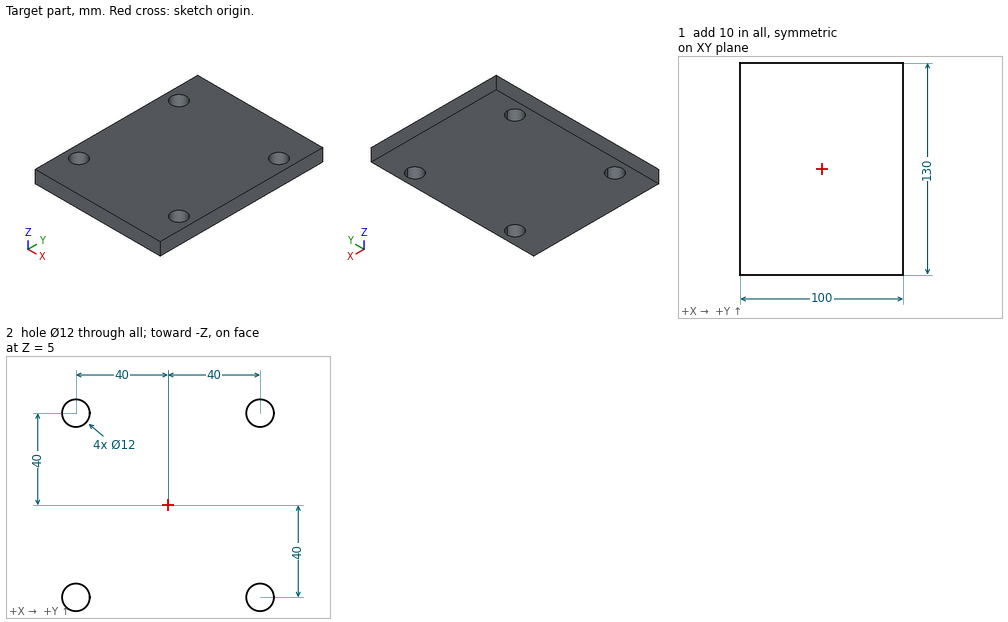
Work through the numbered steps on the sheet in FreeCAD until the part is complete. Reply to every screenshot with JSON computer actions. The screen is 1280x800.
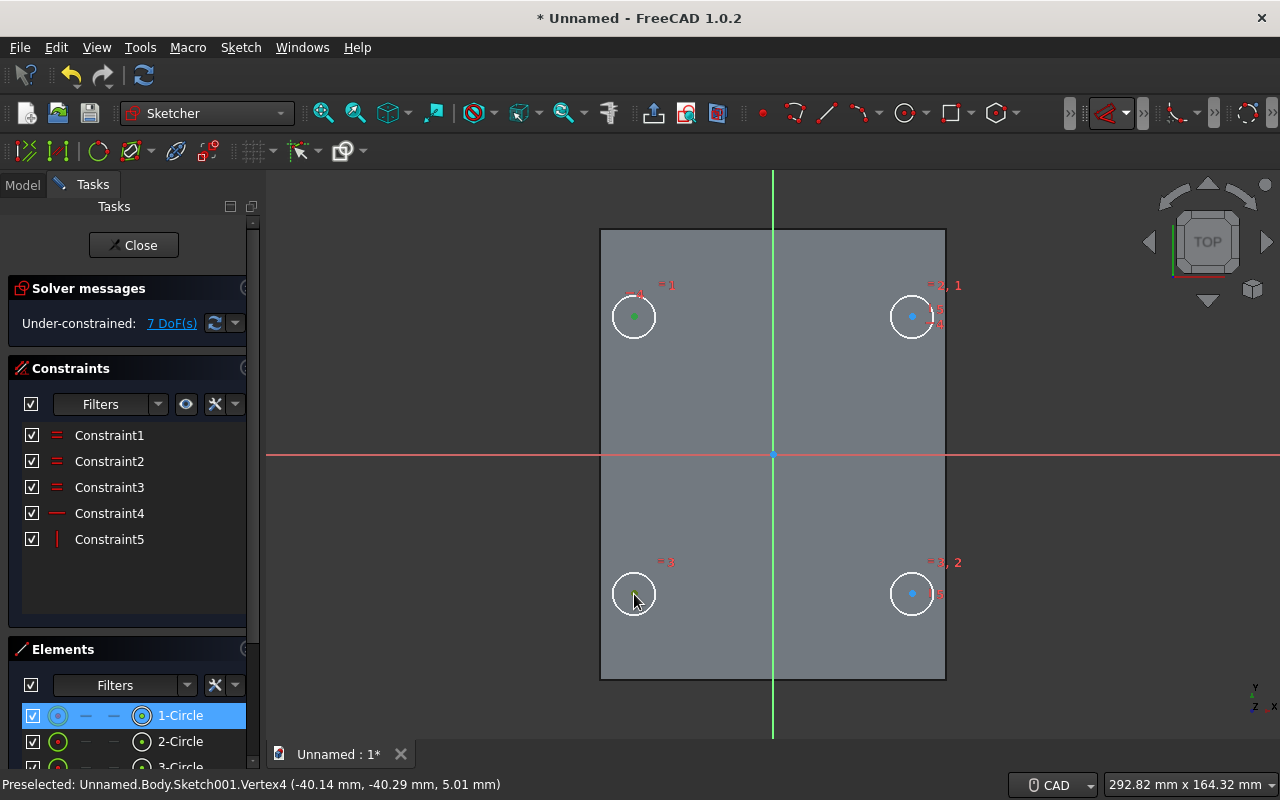
{"action": "key", "text": "v"}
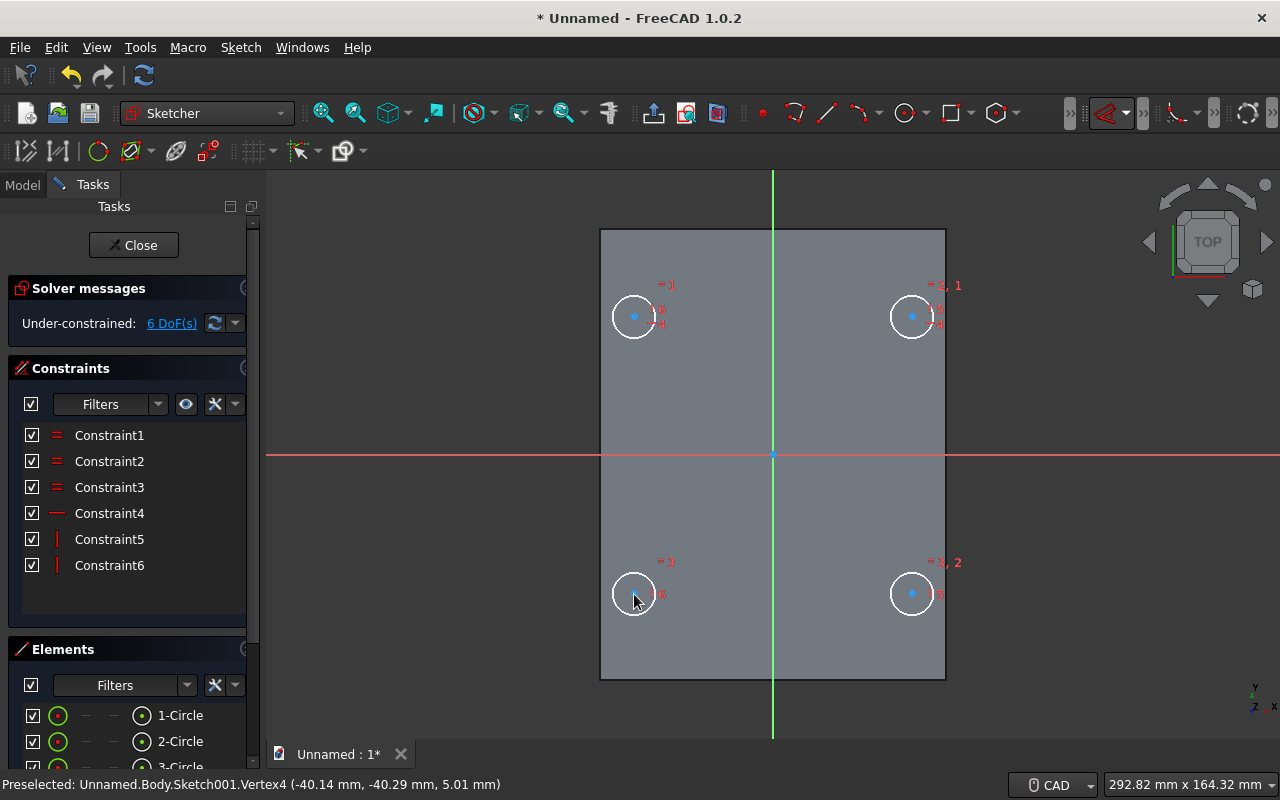
{"action": "left_click", "coordinate": [912, 594]}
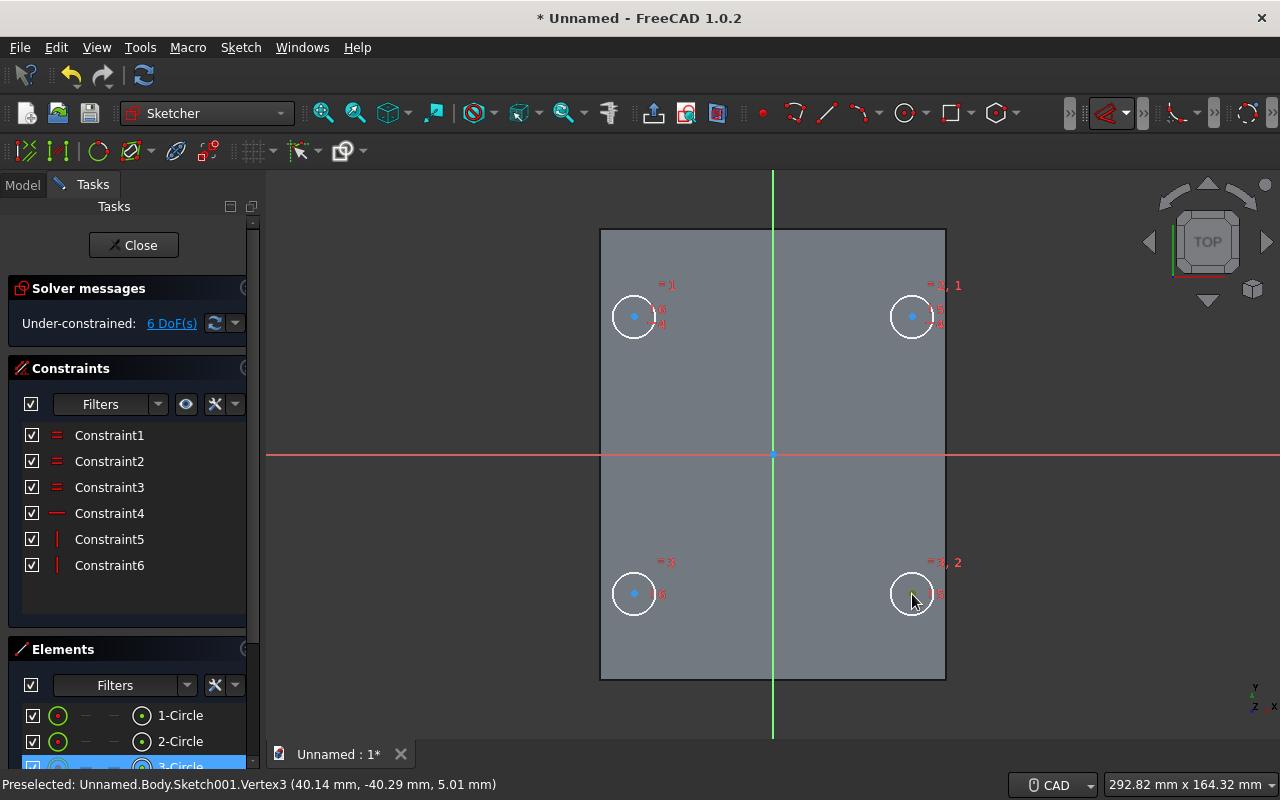
{"action": "left_click", "coordinate": [634, 594]}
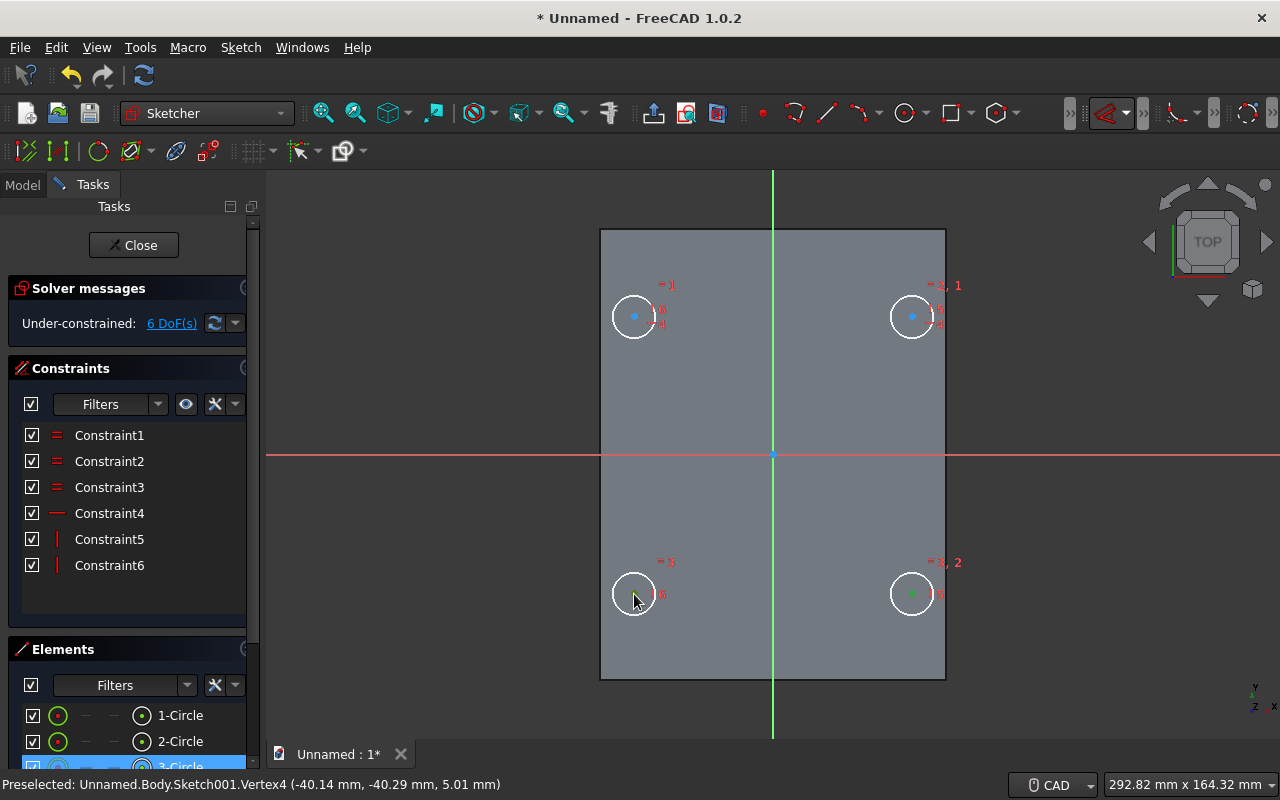
{"action": "key", "text": "h"}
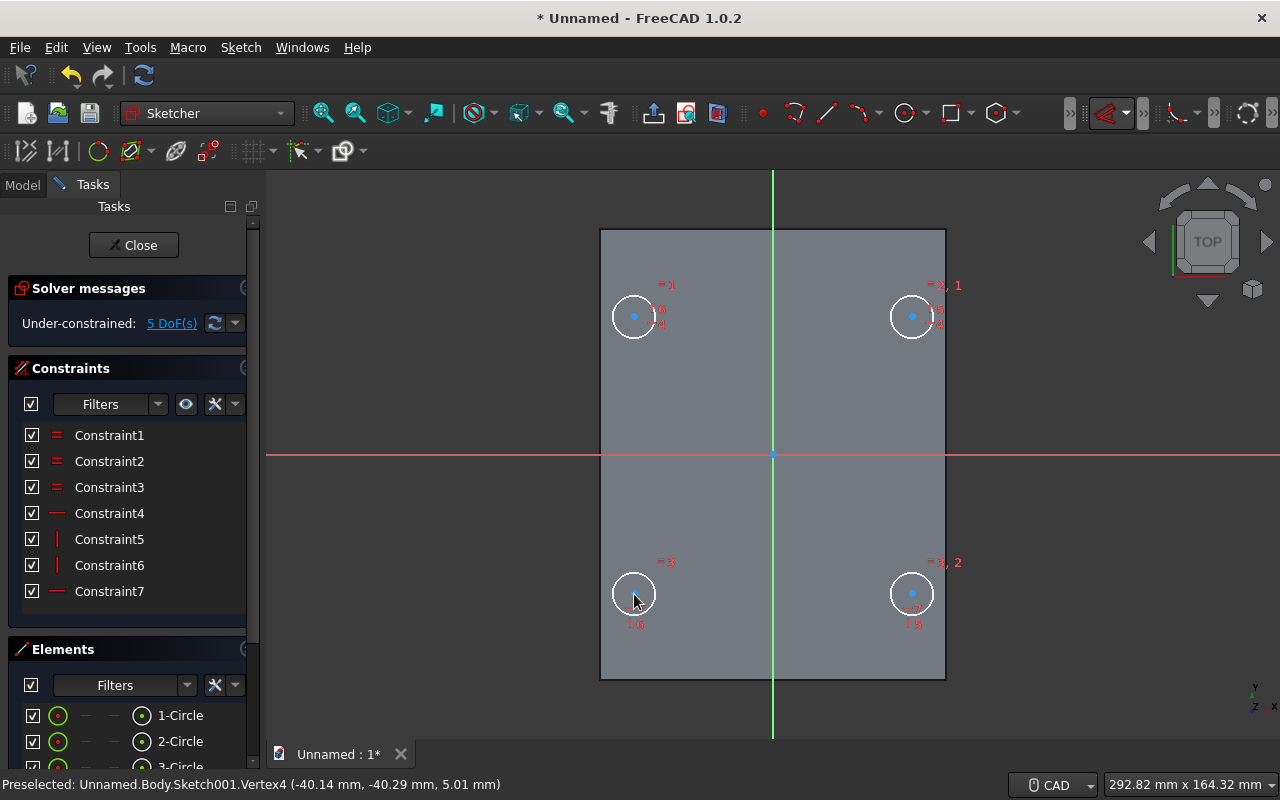
{"action": "left_click", "coordinate": [619, 302]}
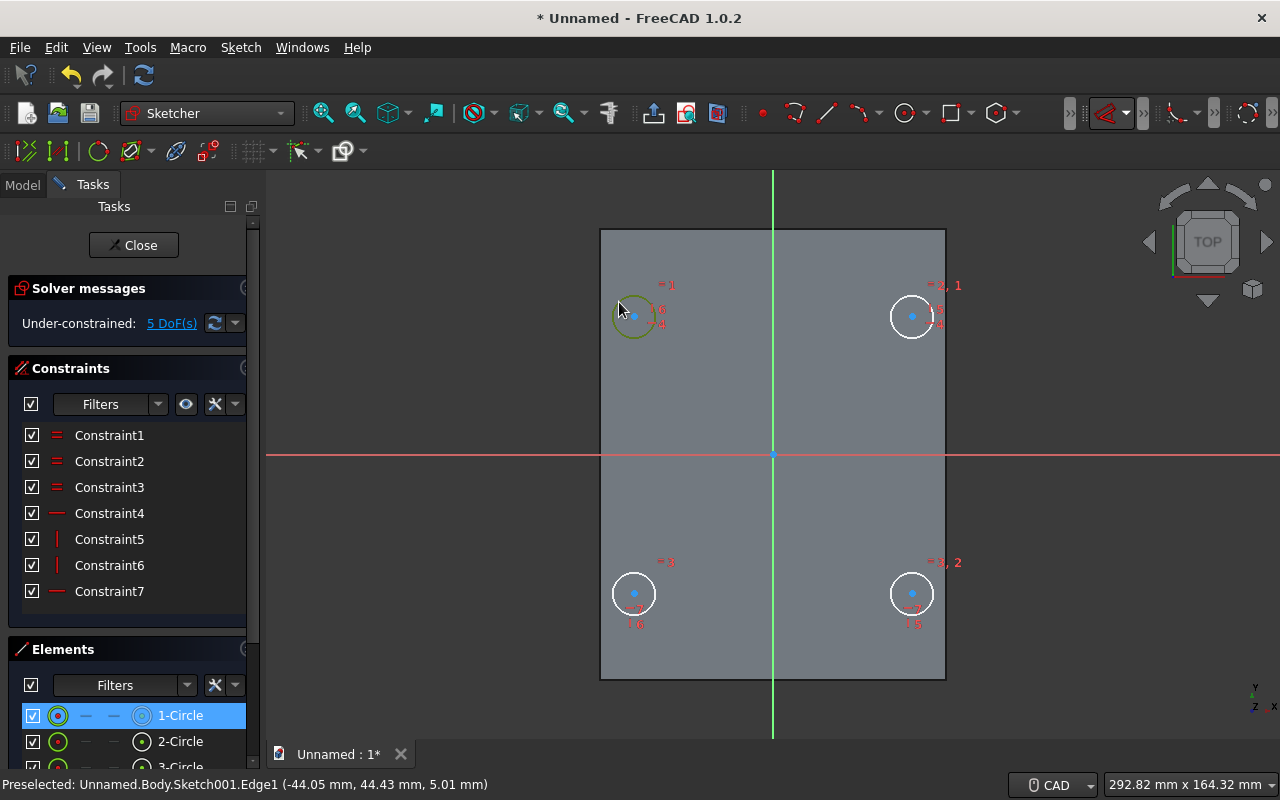
{"action": "left_click", "coordinate": [1128, 114]}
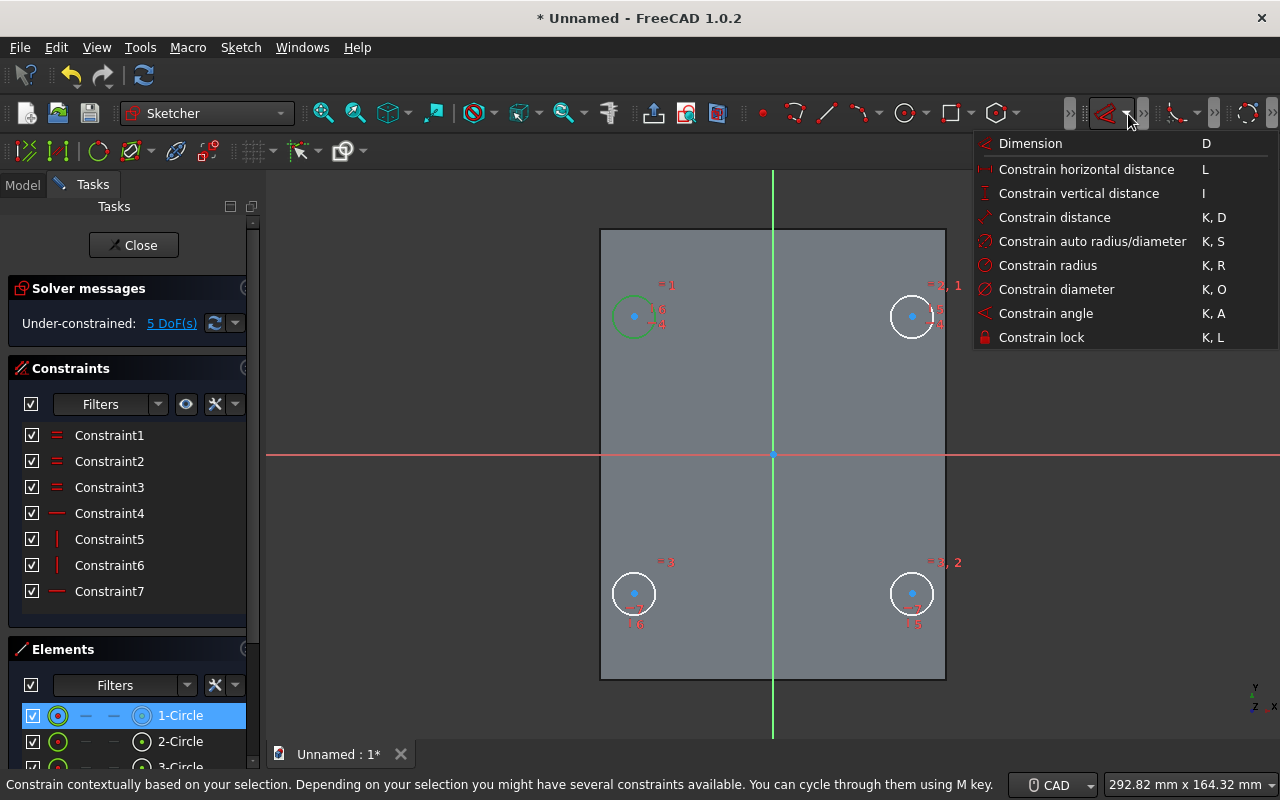
{"action": "left_click", "coordinate": [1126, 289]}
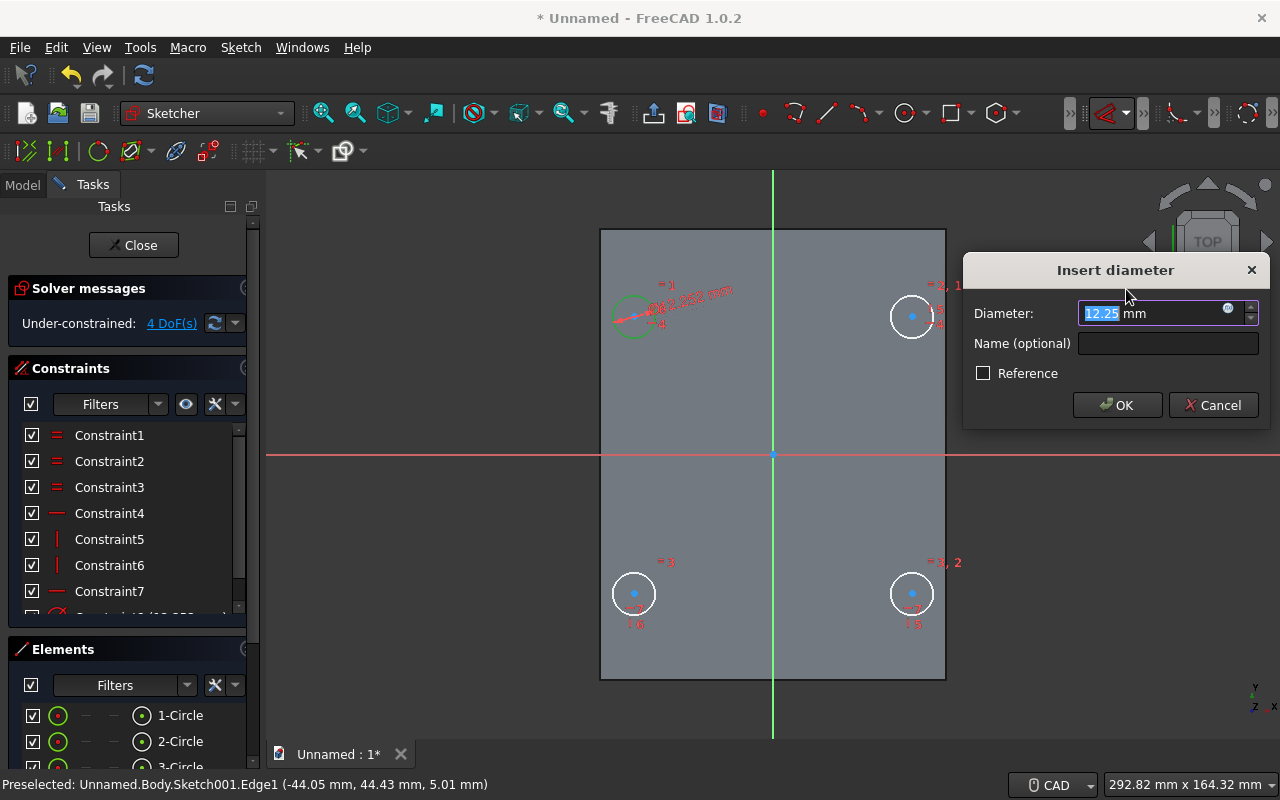
{"action": "type", "text": "12"}
{"action": "key", "text": "Return"}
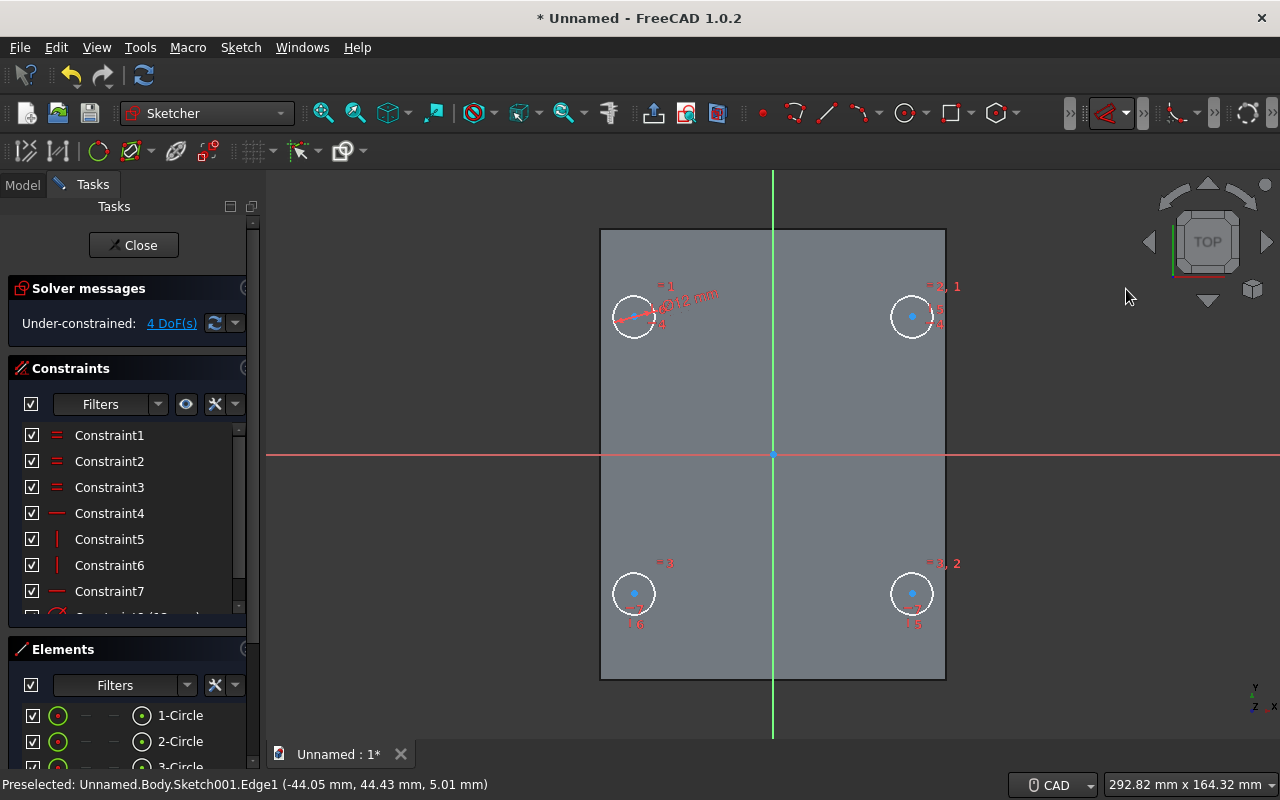
{"action": "left_click", "coordinate": [634, 317]}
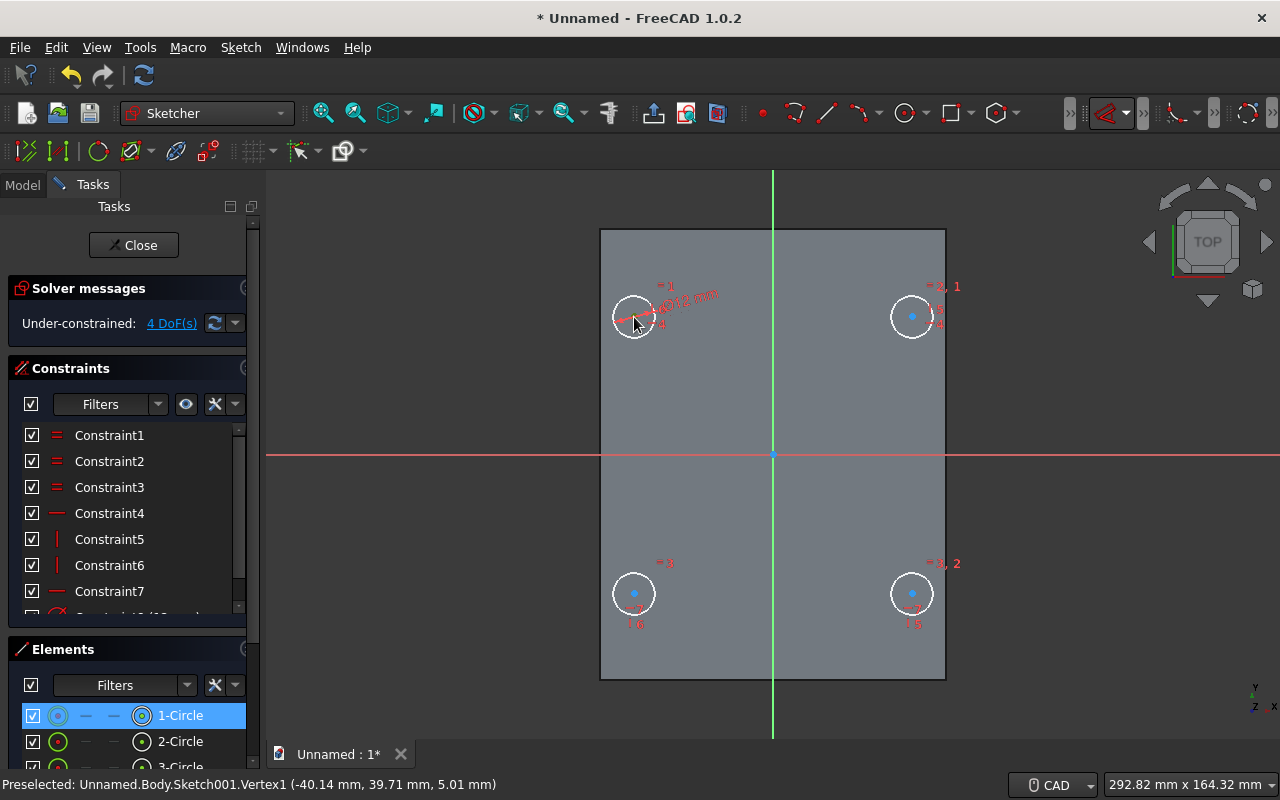
{"action": "key", "text": "l"}